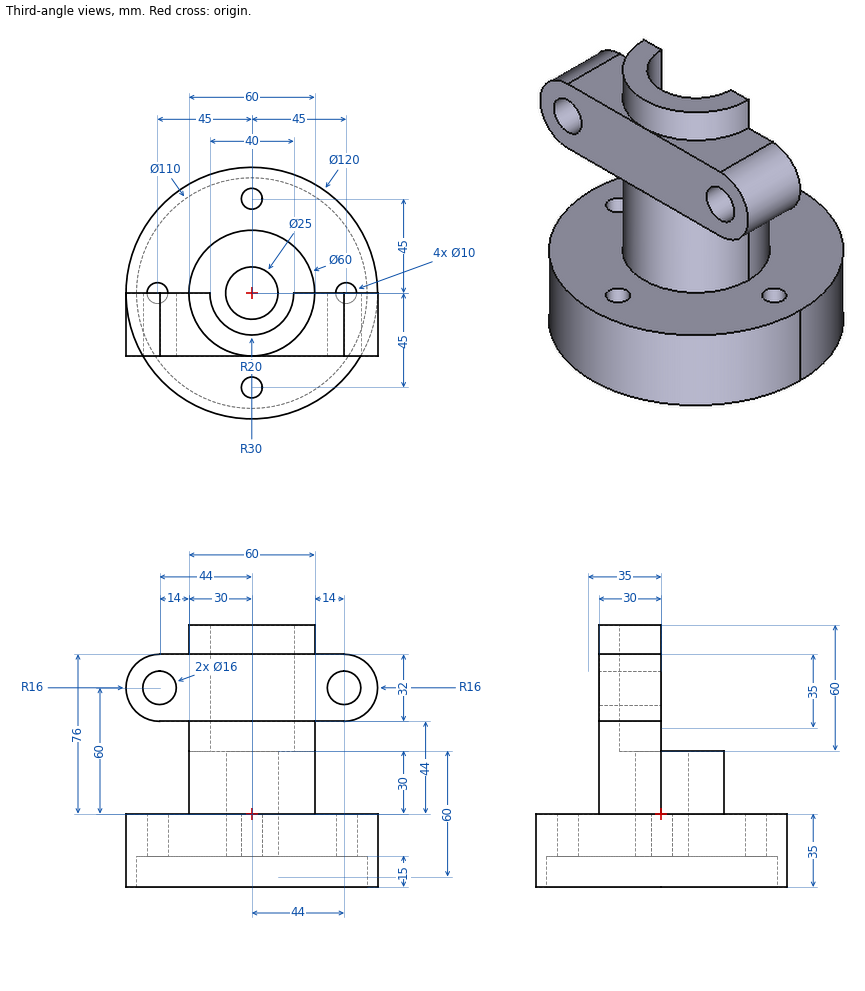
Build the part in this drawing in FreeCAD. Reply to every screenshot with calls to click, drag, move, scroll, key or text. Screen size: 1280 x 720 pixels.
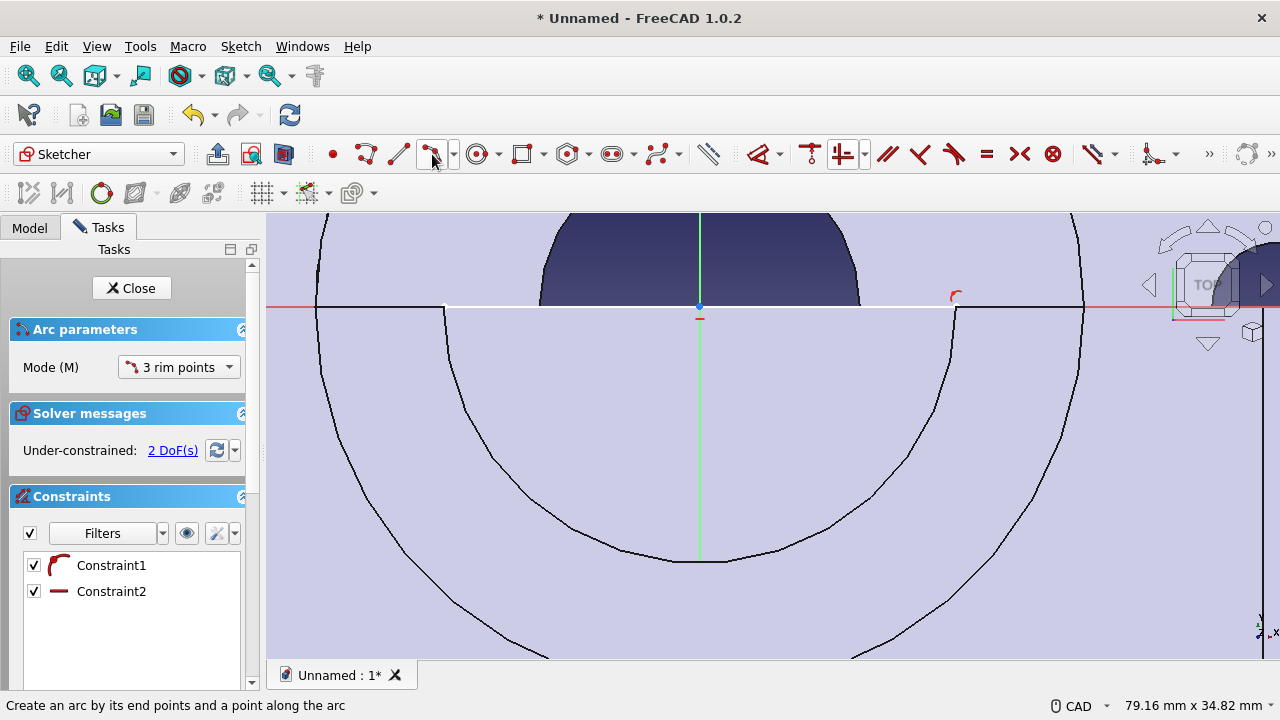
click(444, 316)
click(956, 307)
click(621, 551)
key(Escape)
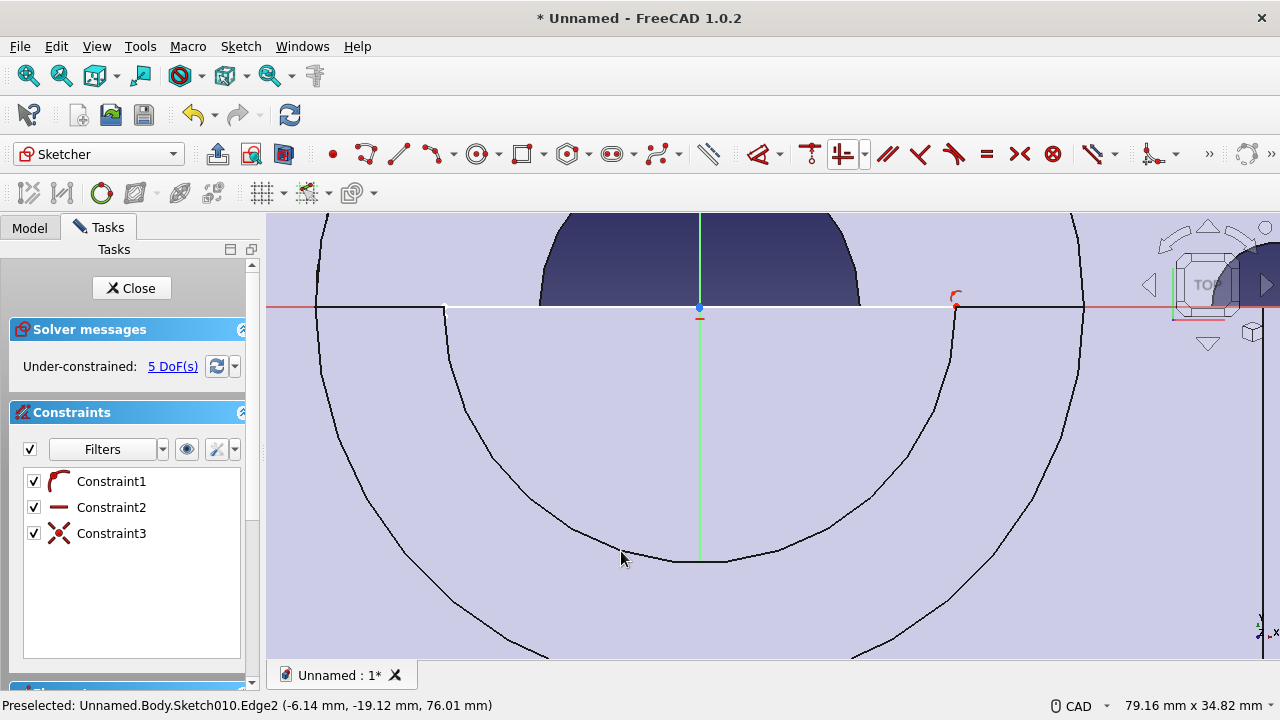
drag(690, 297, 710, 318)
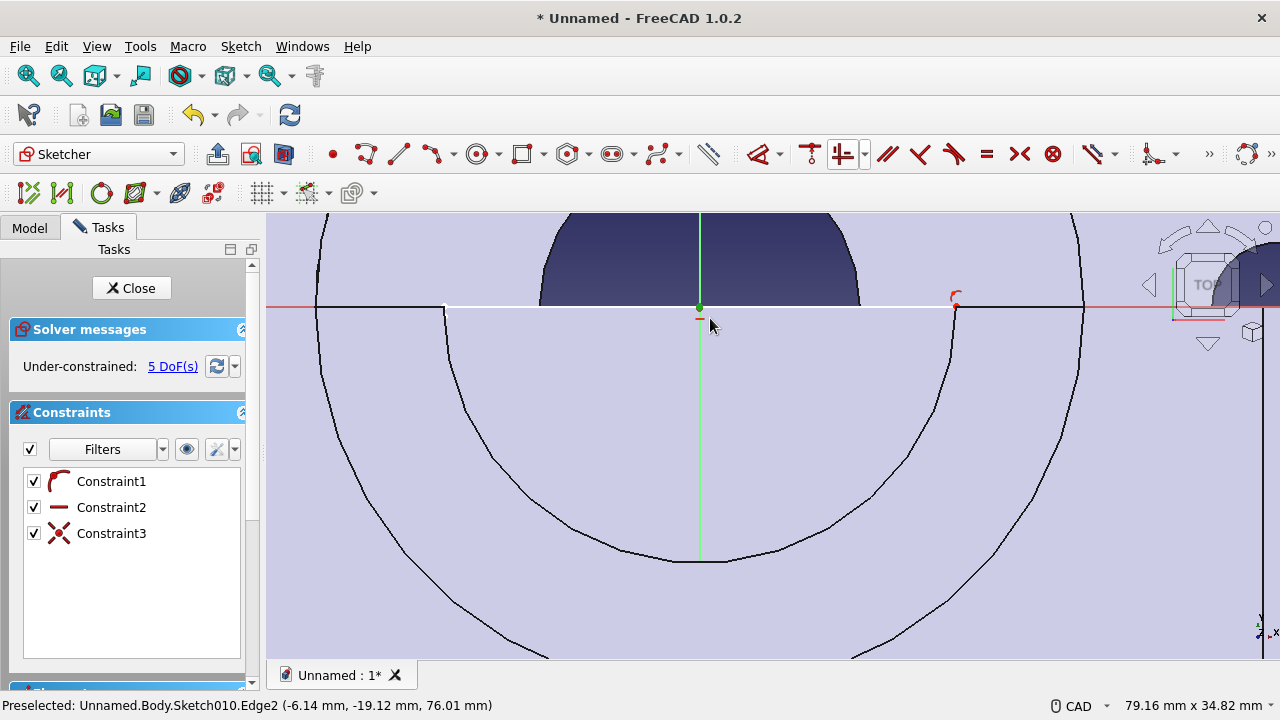
click(810, 154)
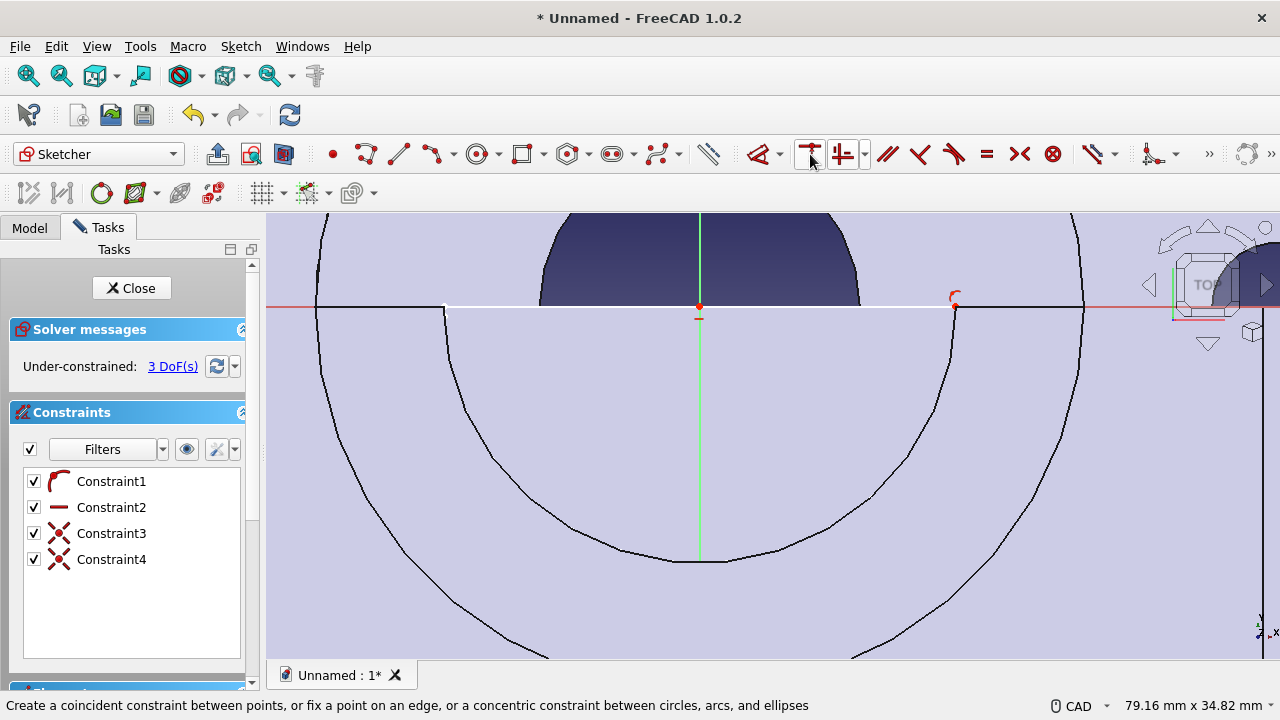
click(758, 154)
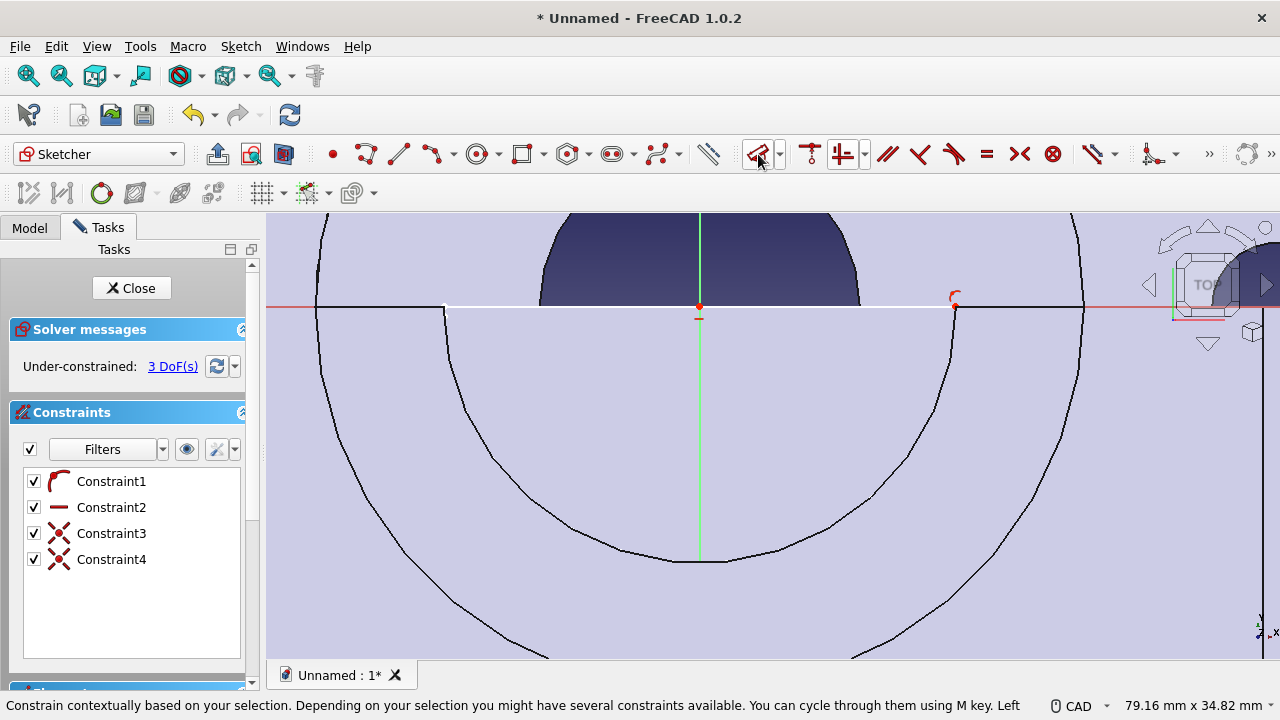
click(555, 518)
click(537, 544)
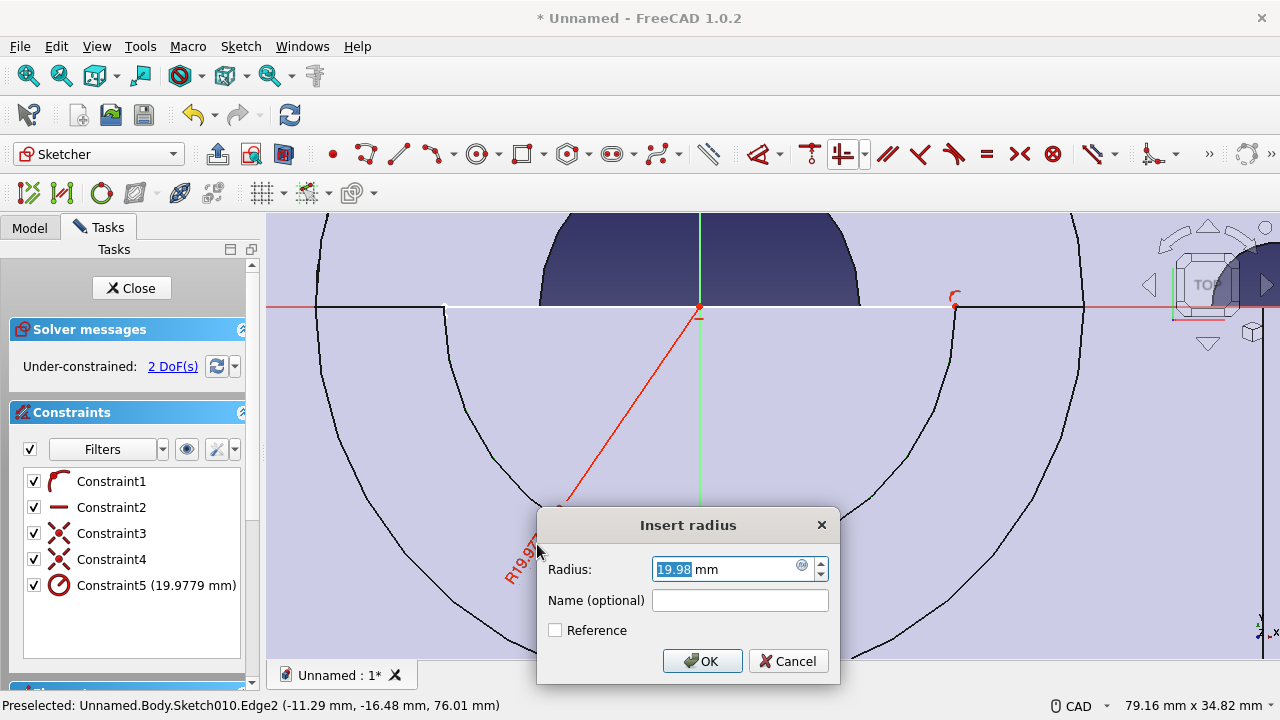
text(20)
key(Return)
key(Escape)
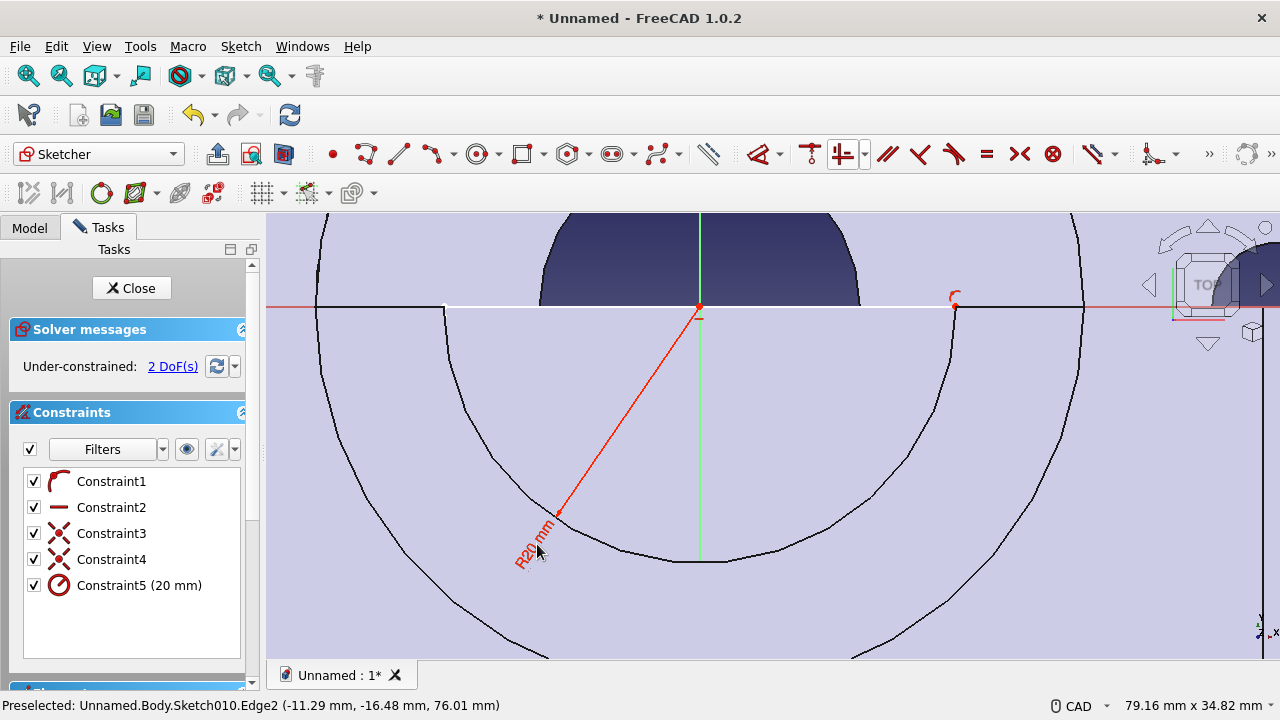
click(444, 317)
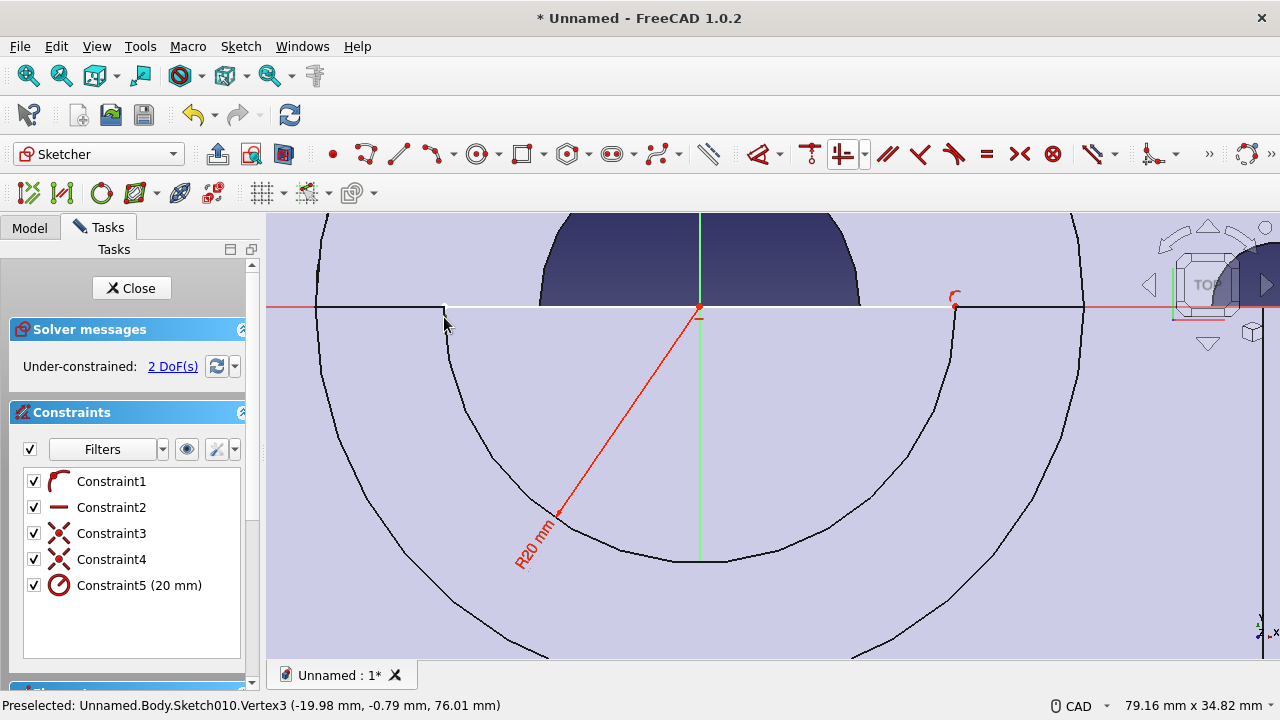
click(353, 307)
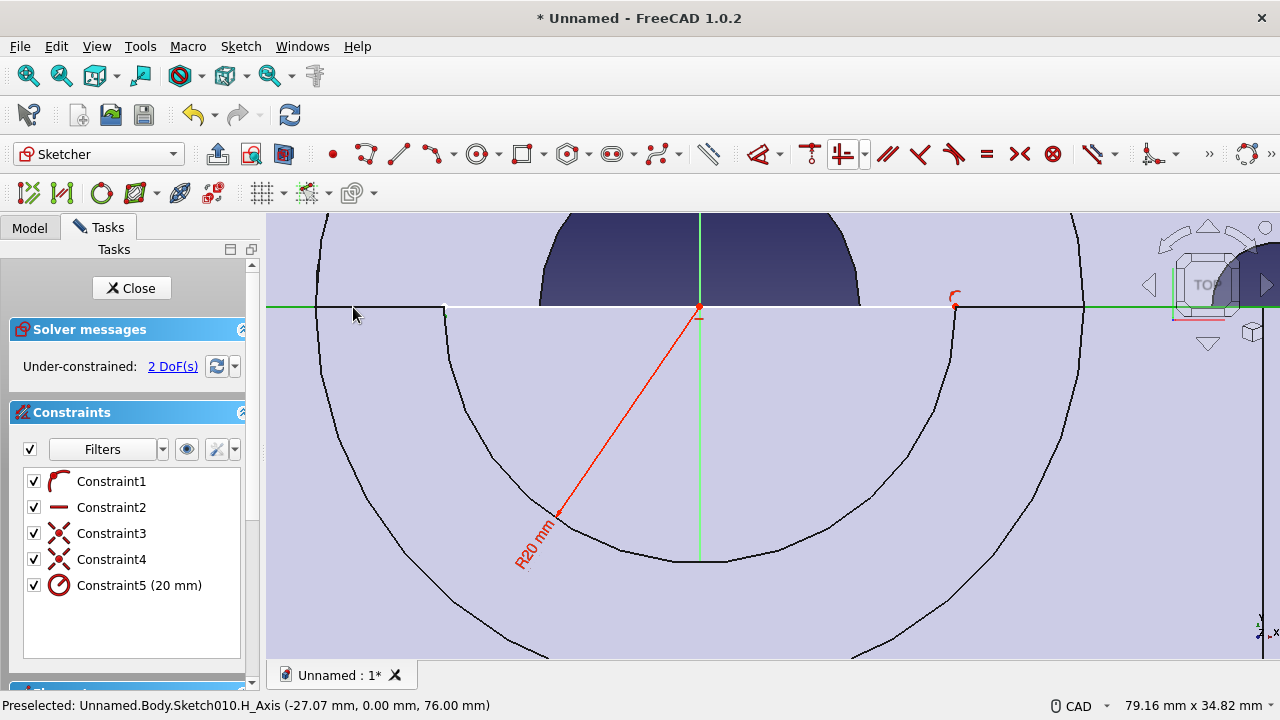
click(810, 154)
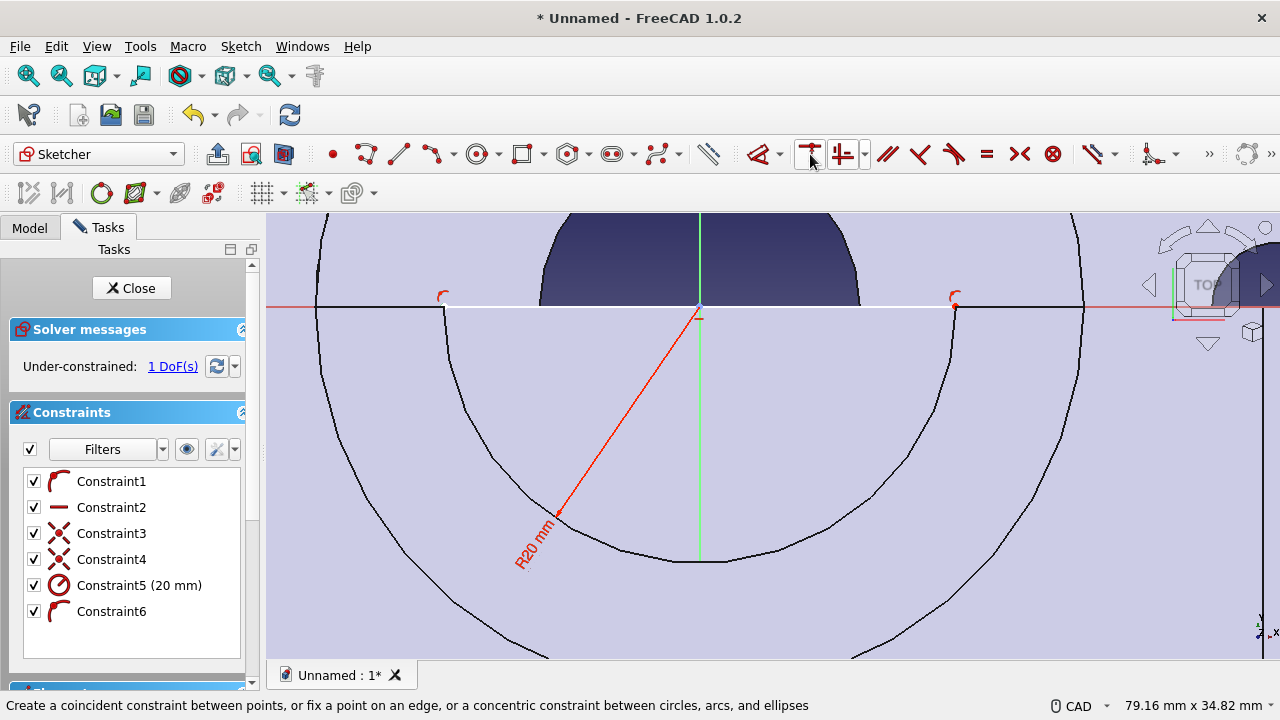
click(758, 154)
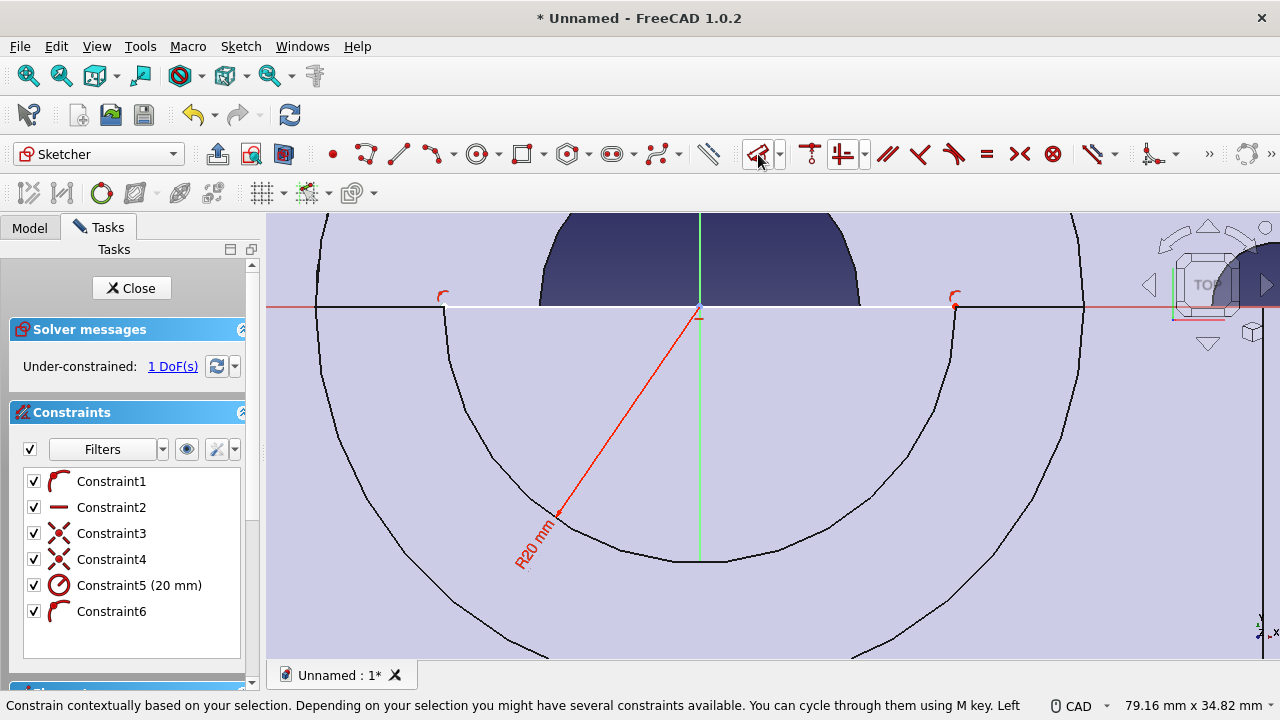
click(802, 307)
click(582, 273)